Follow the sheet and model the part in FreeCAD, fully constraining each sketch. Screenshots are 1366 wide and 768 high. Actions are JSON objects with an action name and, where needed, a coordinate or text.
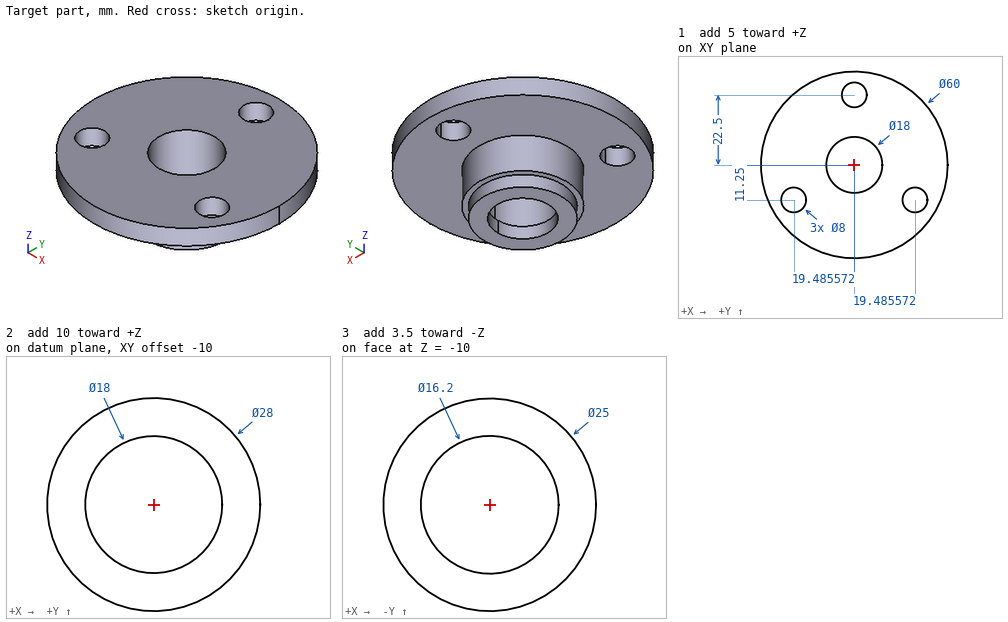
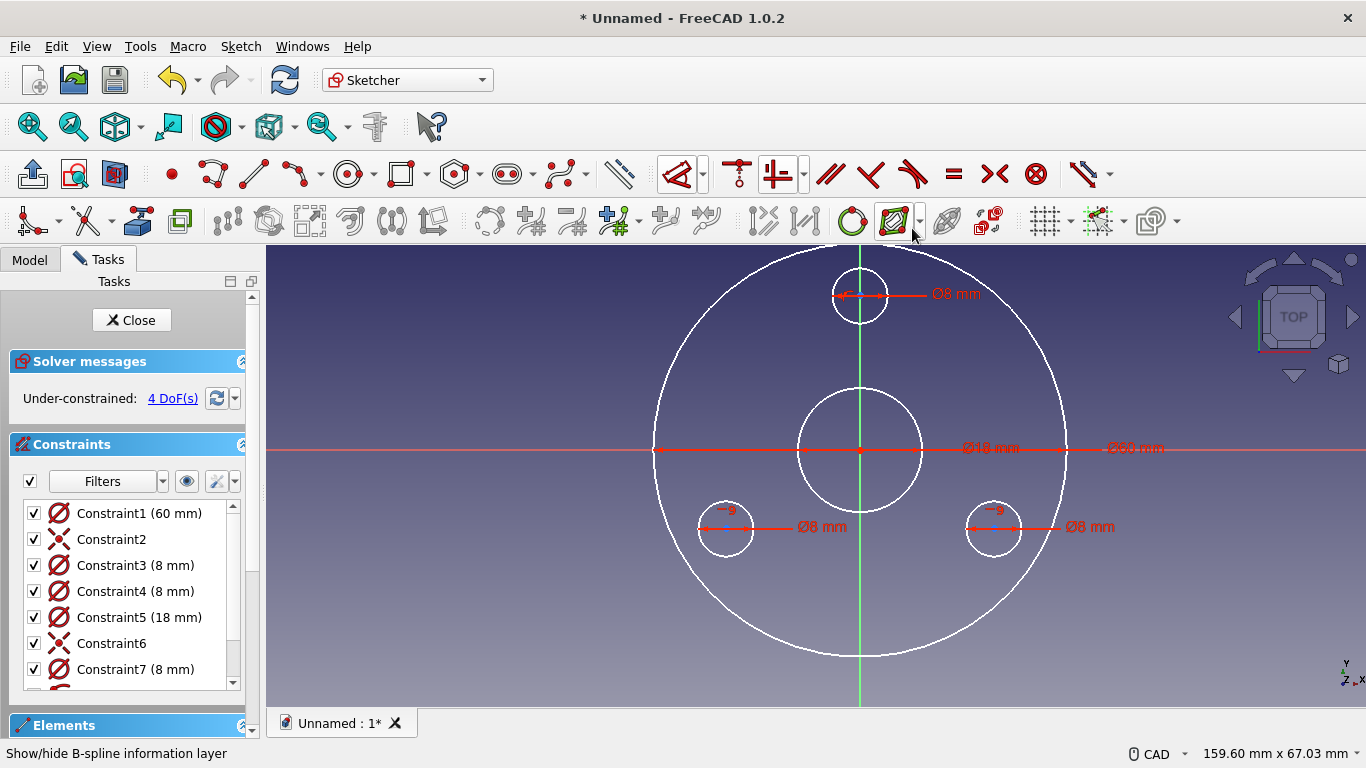
{"action": "key", "text": "d"}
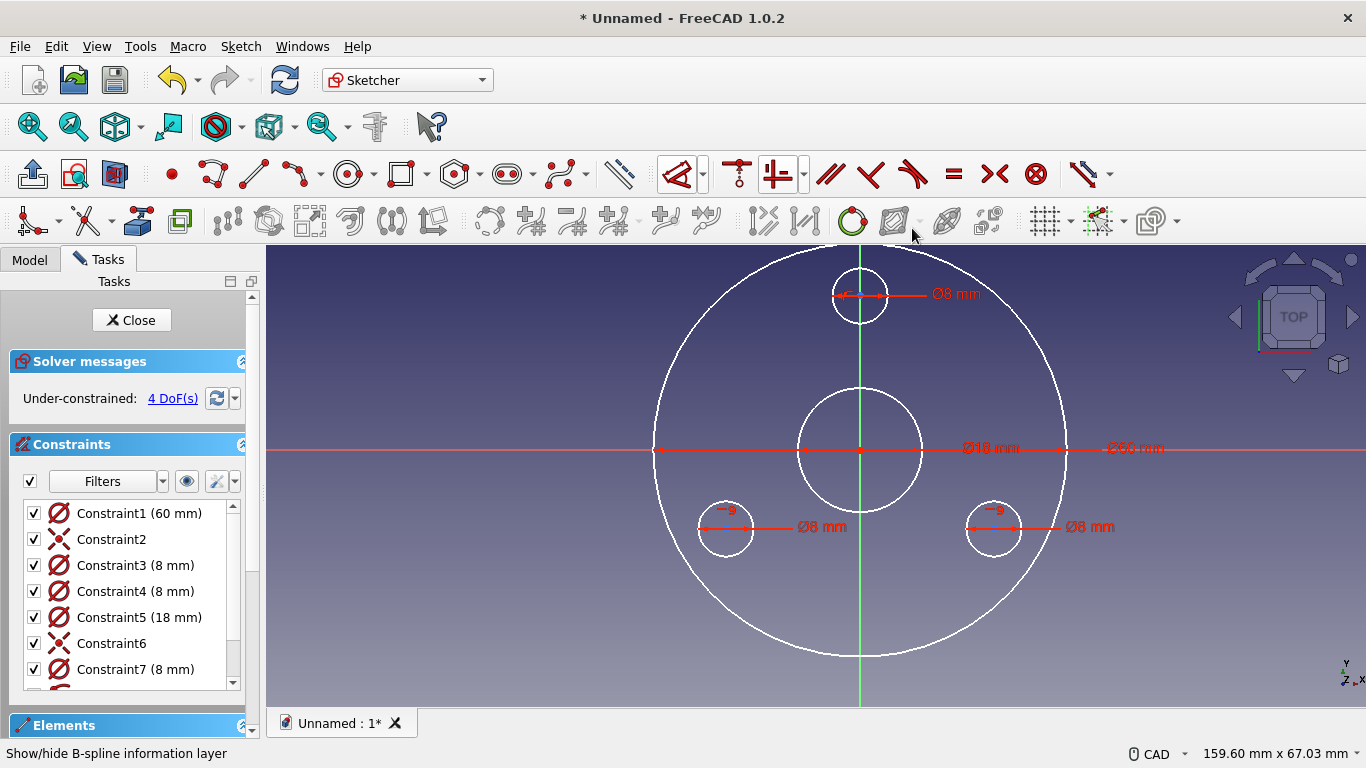
{"action": "left_click", "coordinate": [860, 296]}
{"action": "left_click", "coordinate": [894, 373]}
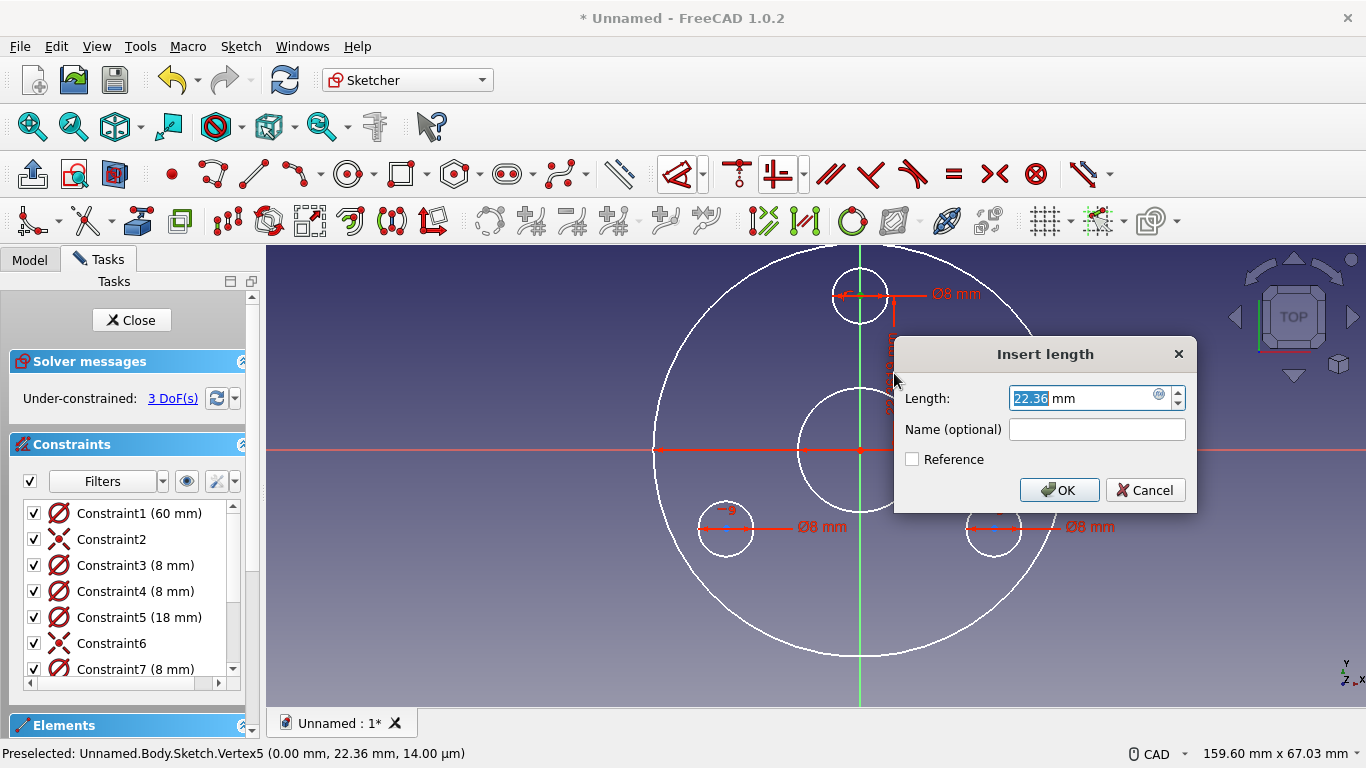
{"action": "type", "text": "22.5"}
{"action": "key", "text": "Return"}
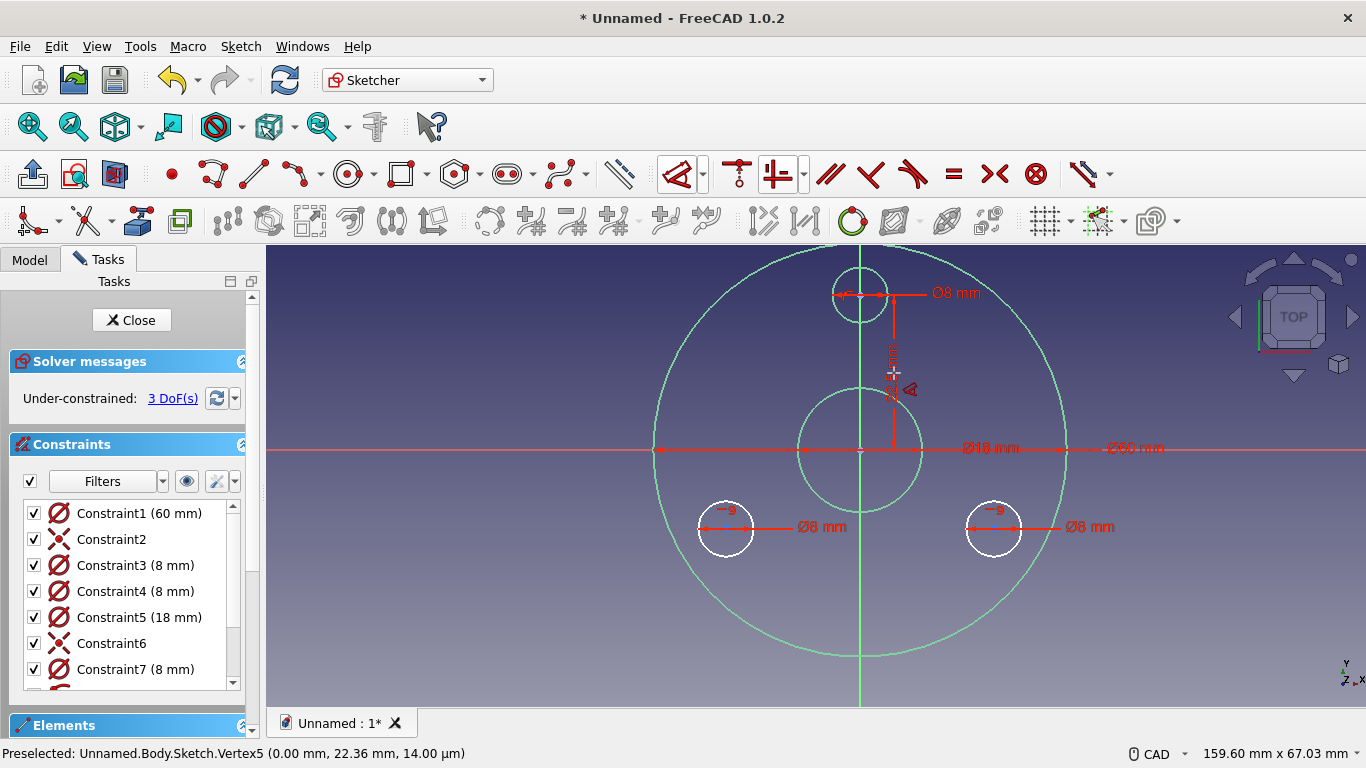
{"action": "left_click", "coordinate": [726, 529]}
{"action": "left_click", "coordinate": [692, 490]}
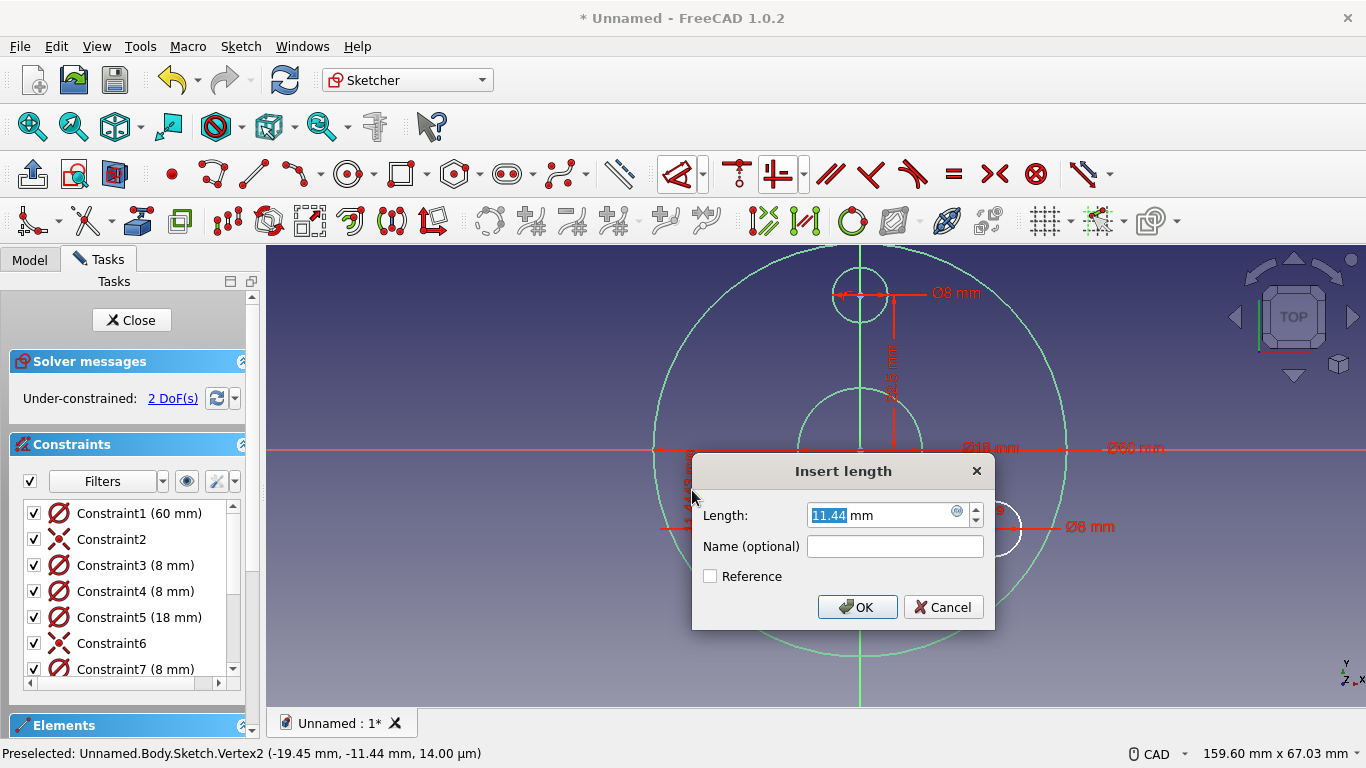
{"action": "type", "text": "11.25"}
{"action": "key", "text": "Return"}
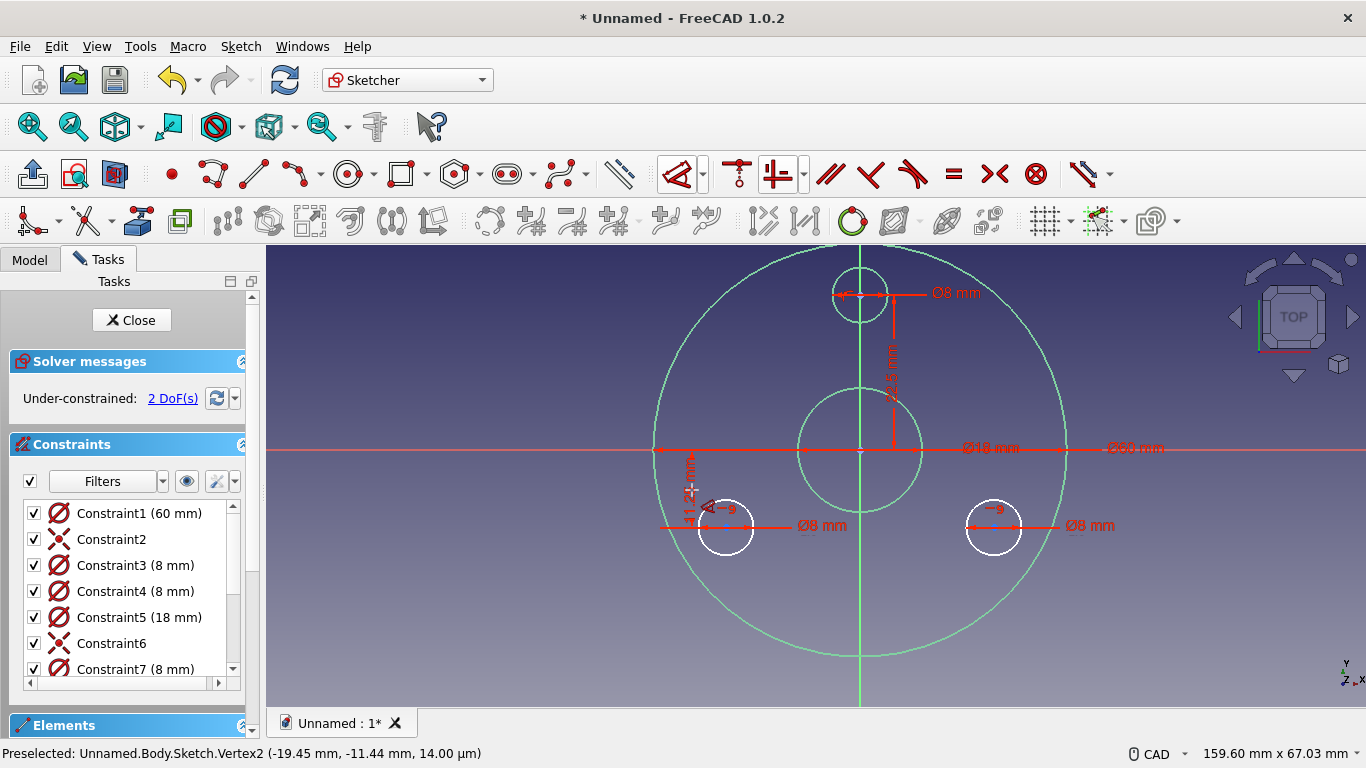
{"action": "left_click", "coordinate": [726, 528]}
{"action": "left_click", "coordinate": [793, 562]}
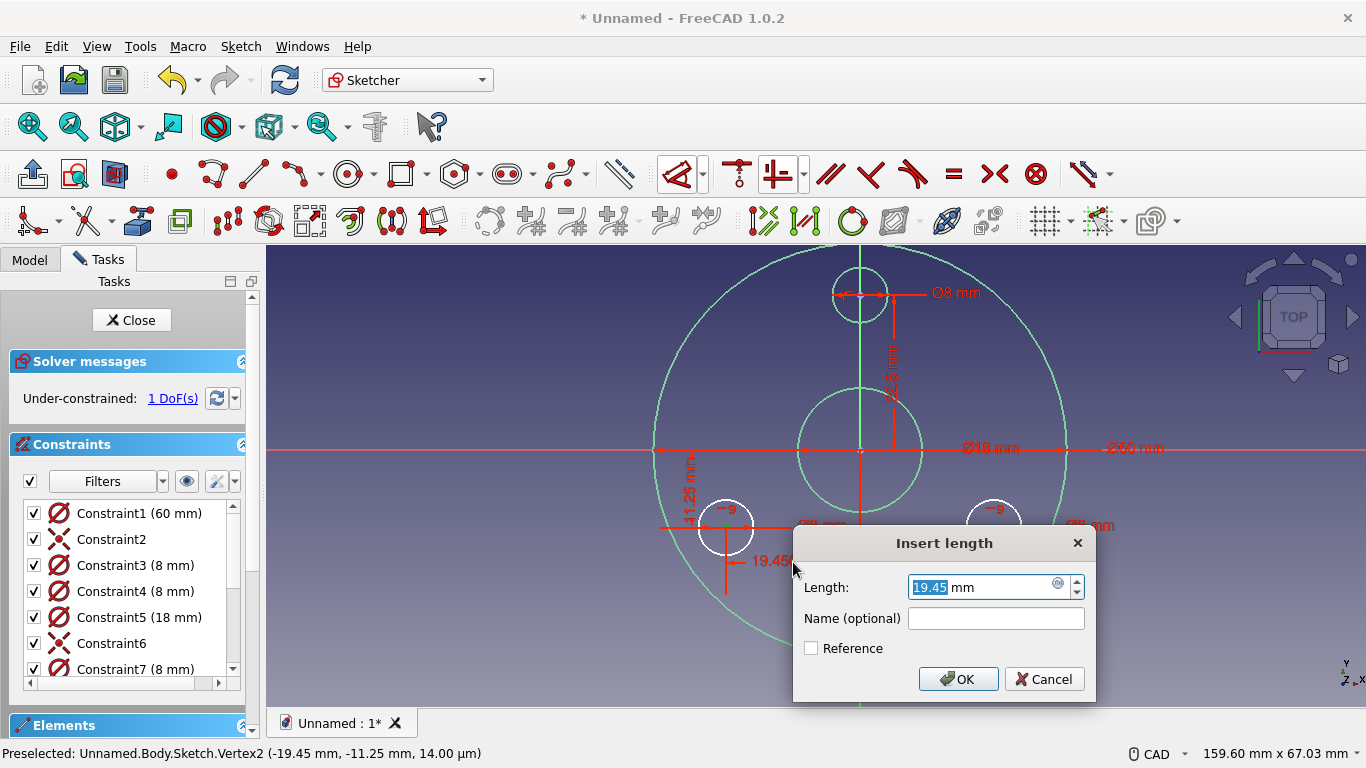
{"action": "type", "text": "19.485572"}
{"action": "key", "text": "Return"}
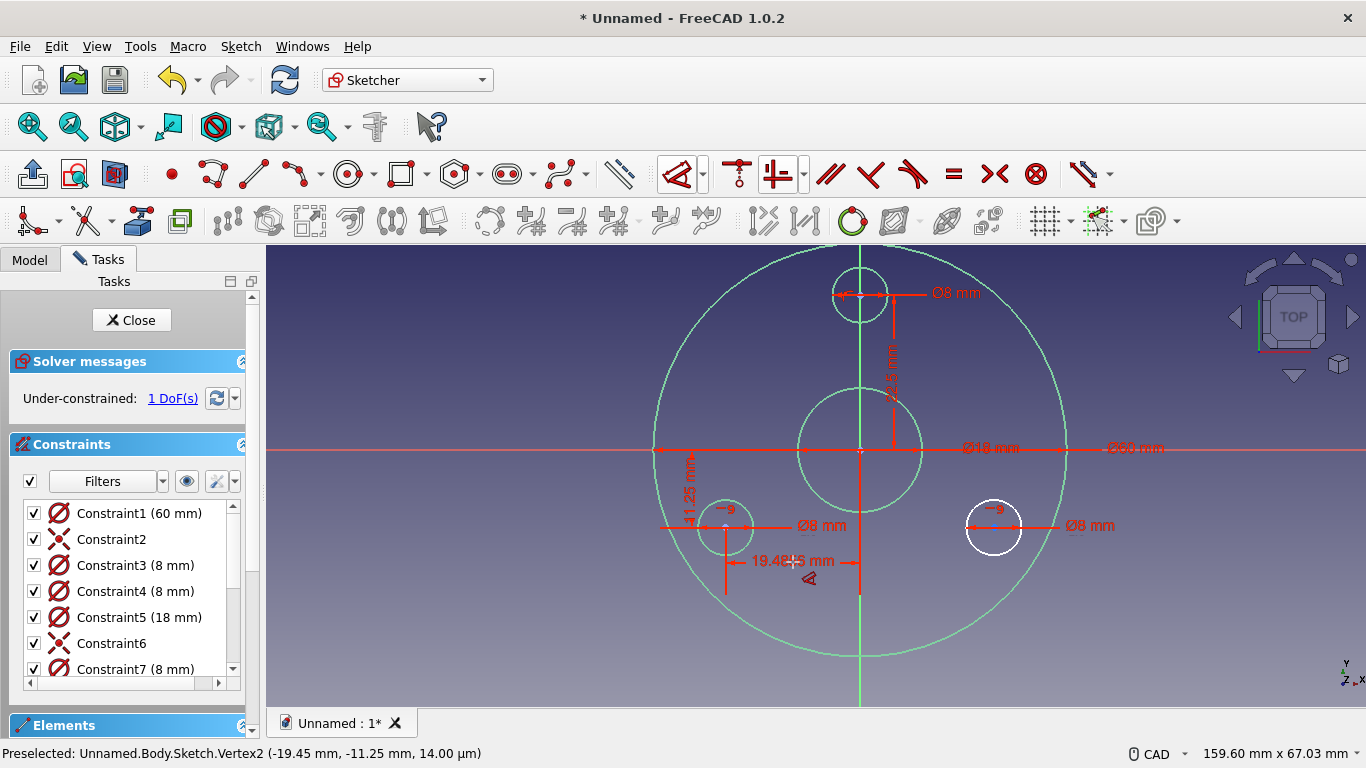
{"action": "left_click", "coordinate": [994, 528]}
{"action": "left_click", "coordinate": [927, 562]}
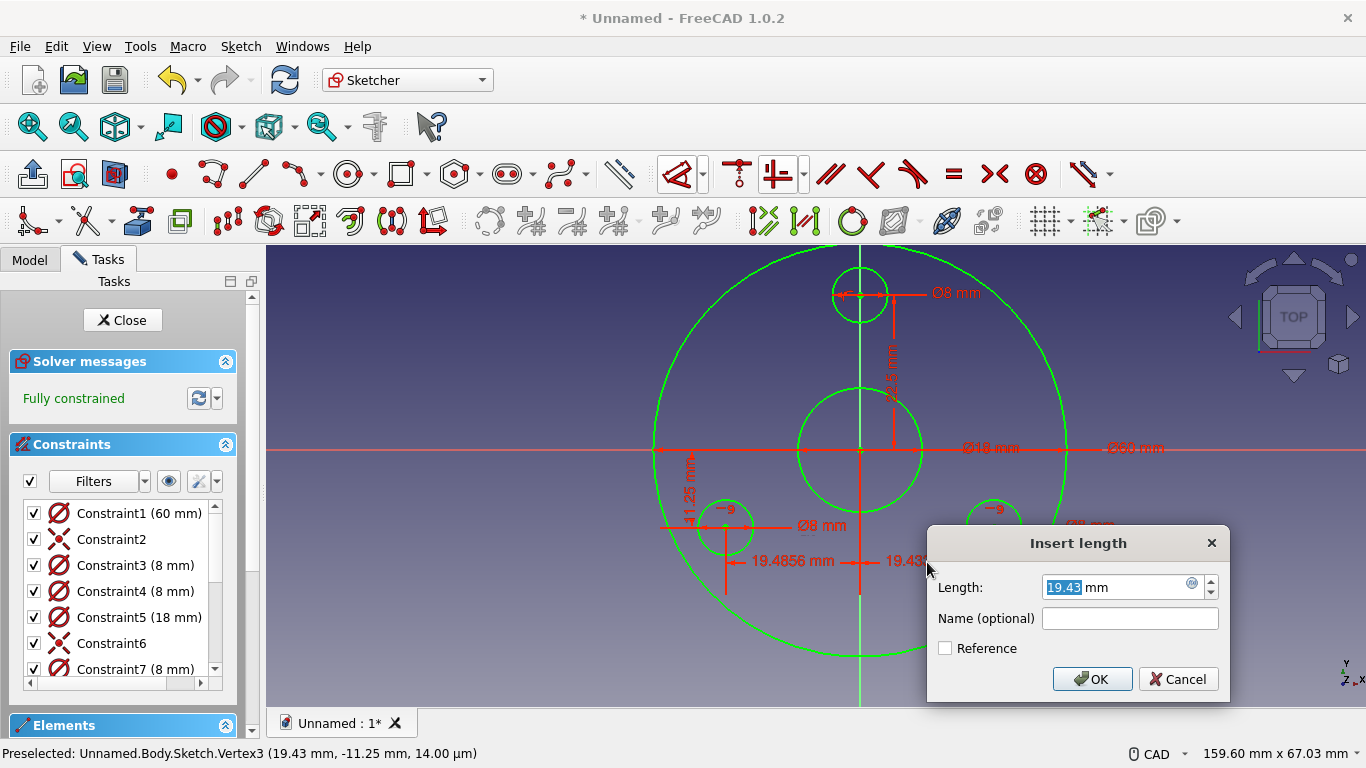
{"action": "type", "text": "19.485572"}
{"action": "key", "text": "Return"}
{"action": "key", "text": "Escape"}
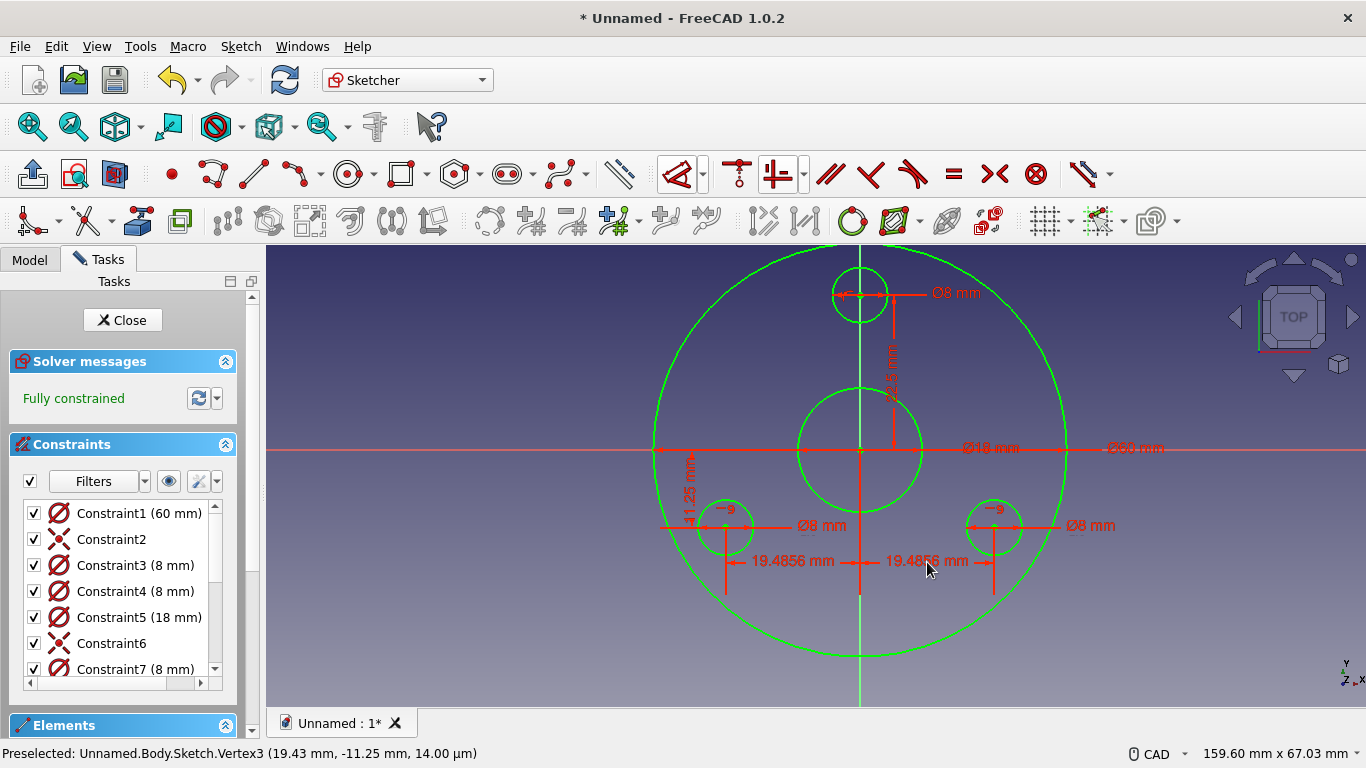
{"action": "left_click", "coordinate": [123, 320]}